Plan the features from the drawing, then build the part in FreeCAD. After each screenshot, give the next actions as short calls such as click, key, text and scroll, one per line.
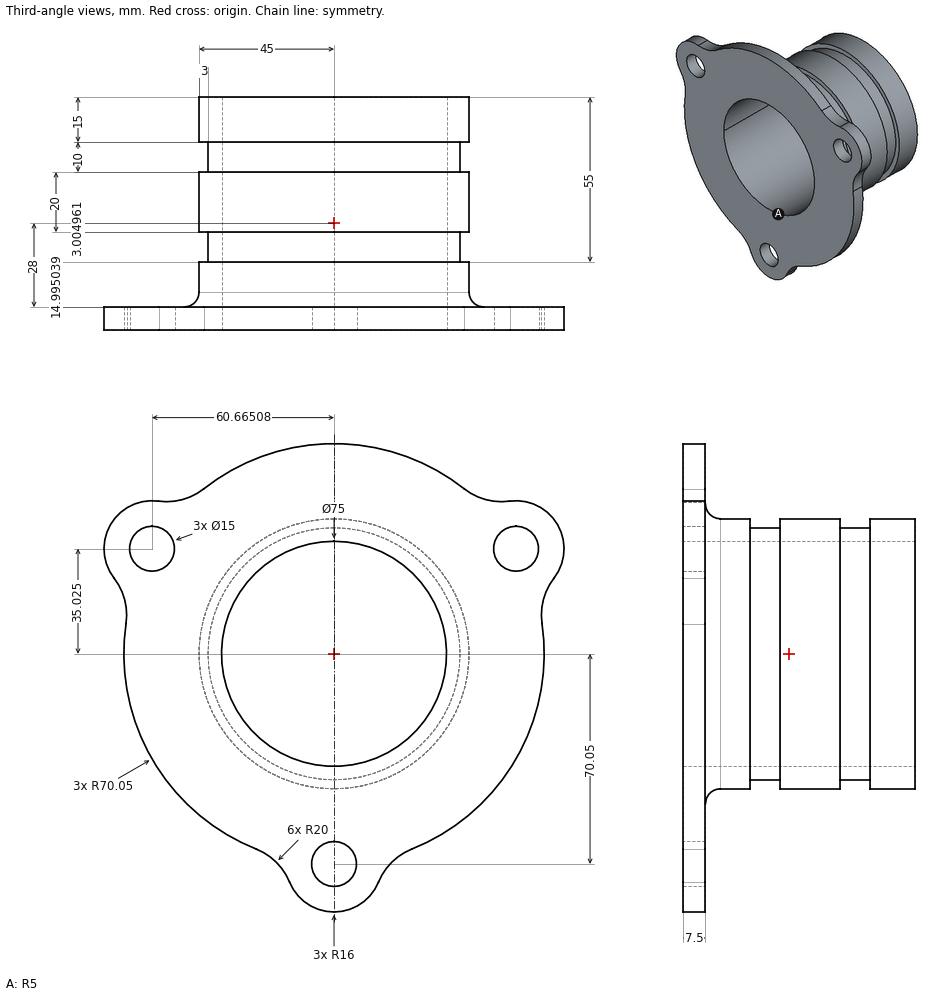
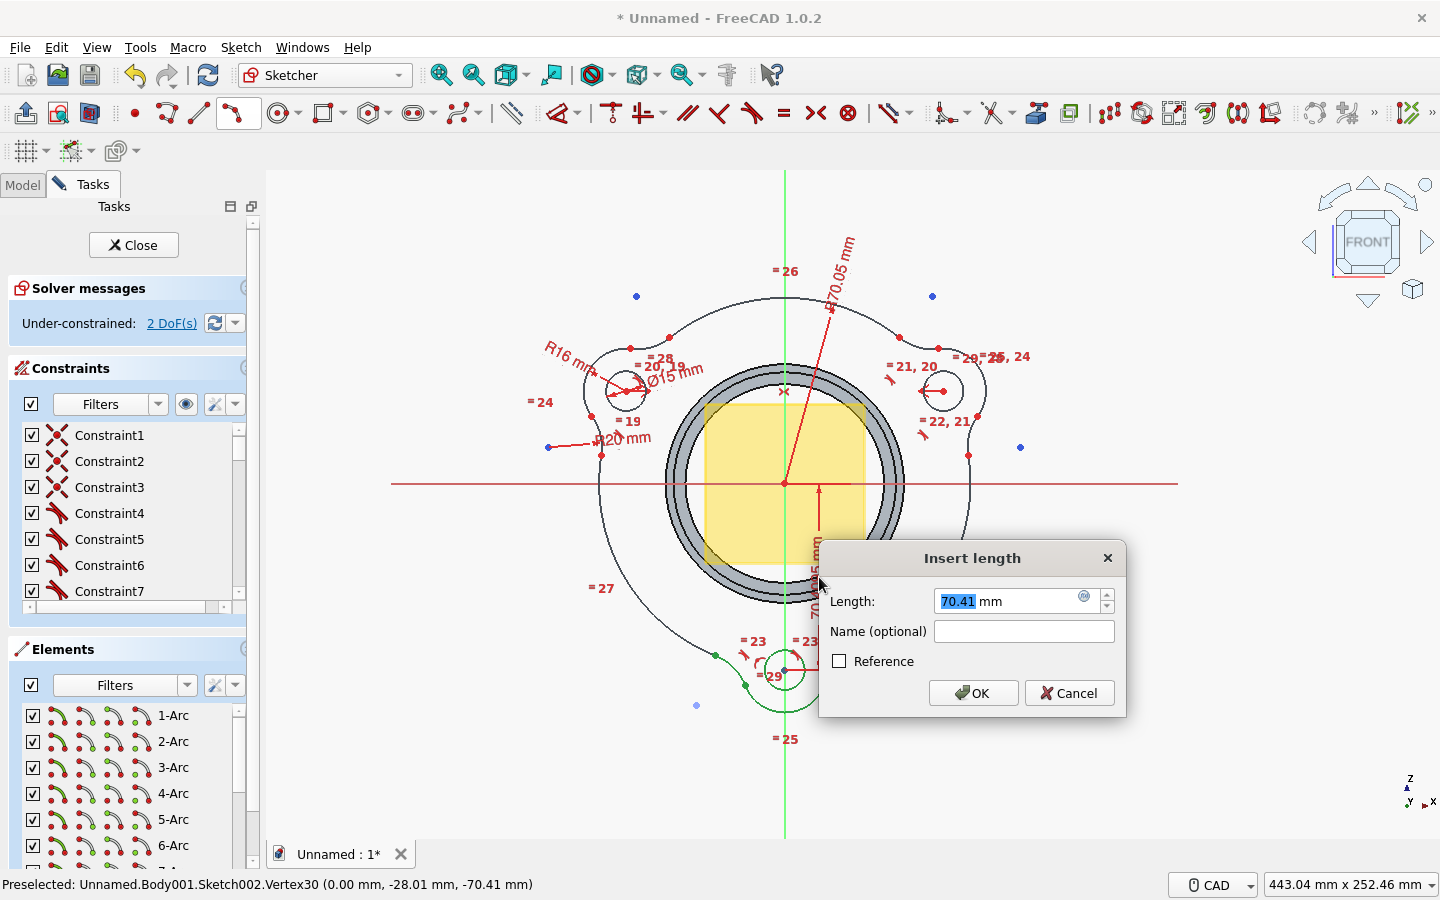
text(70.05)
key(Return)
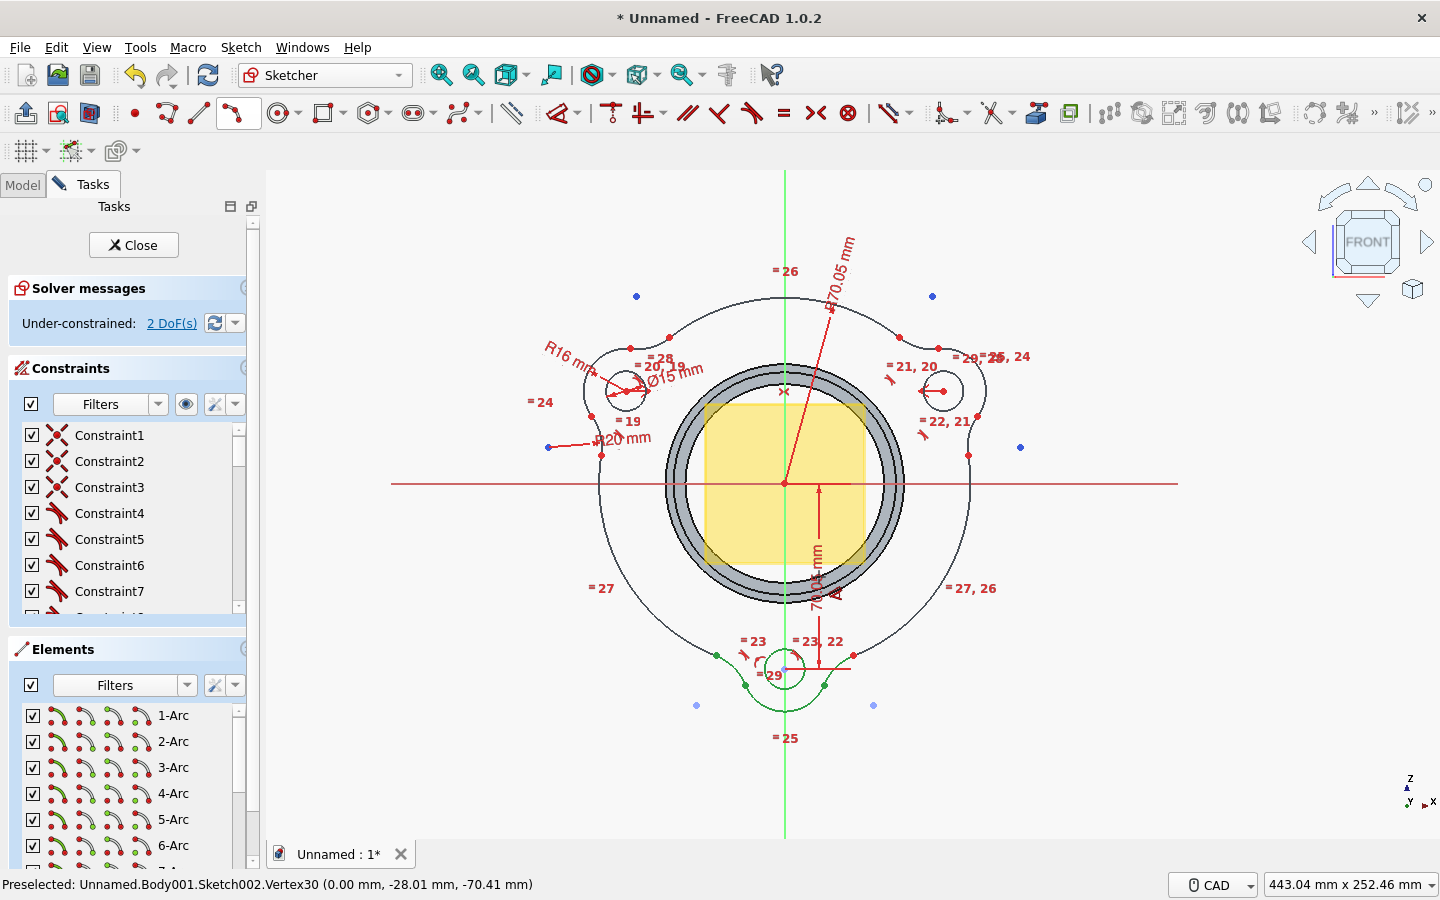
click(626, 391)
click(819, 437)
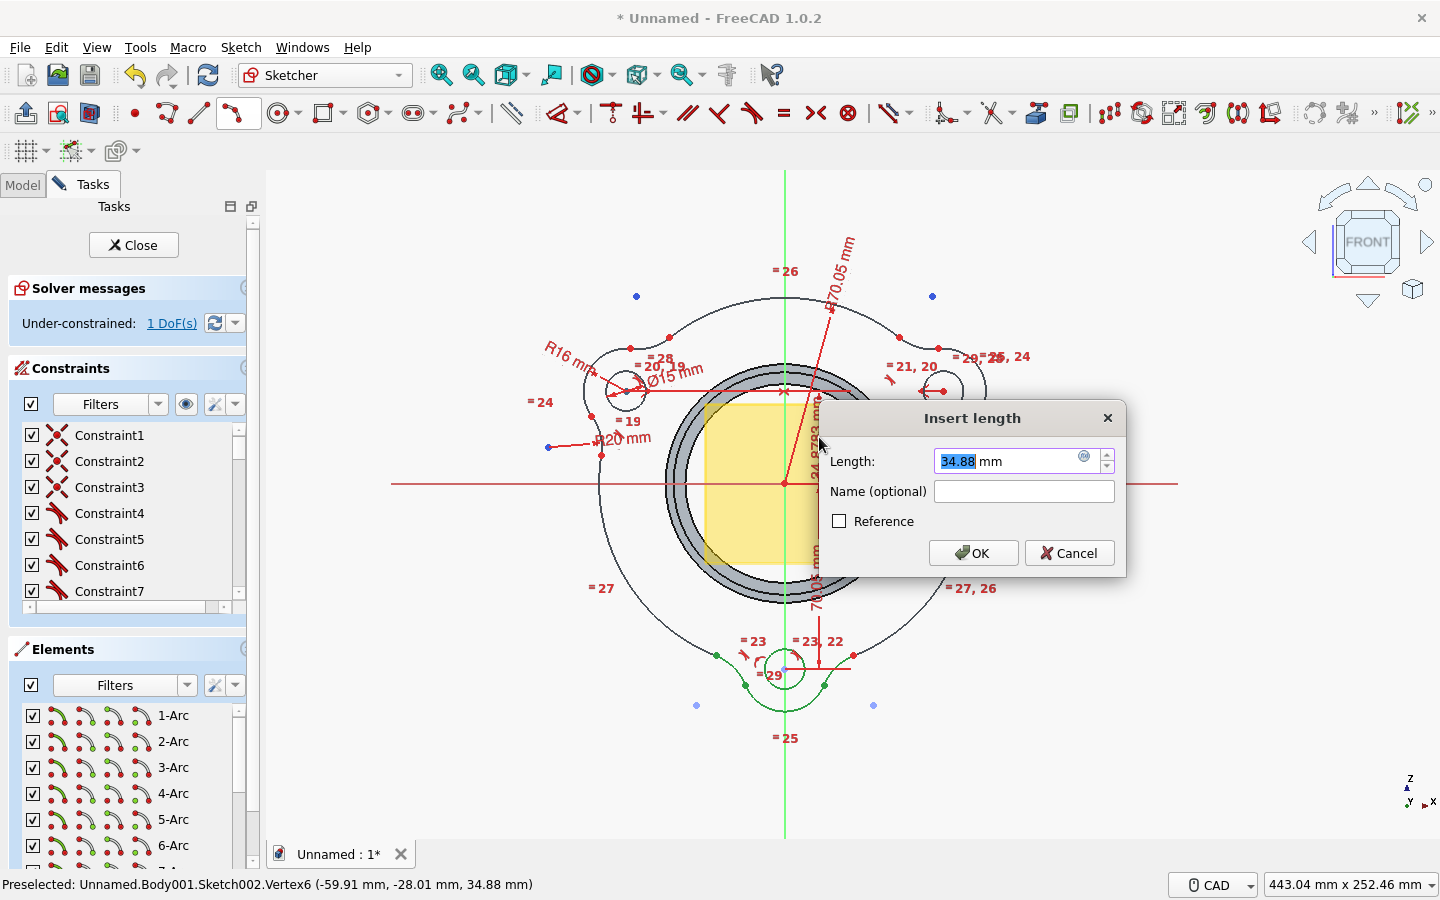
text(35.025)
key(Return)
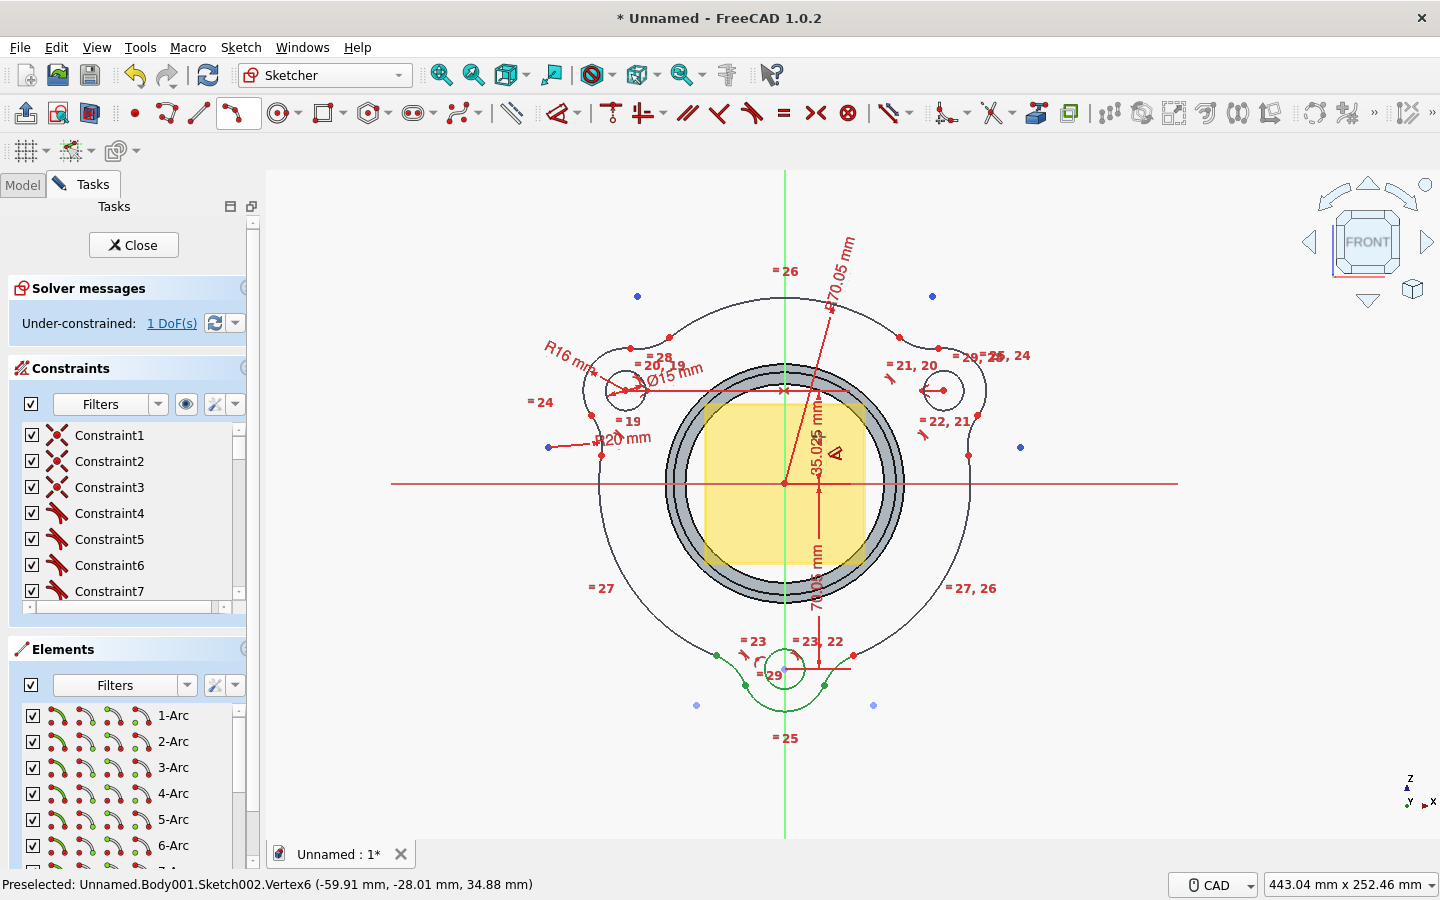
click(626, 391)
click(761, 357)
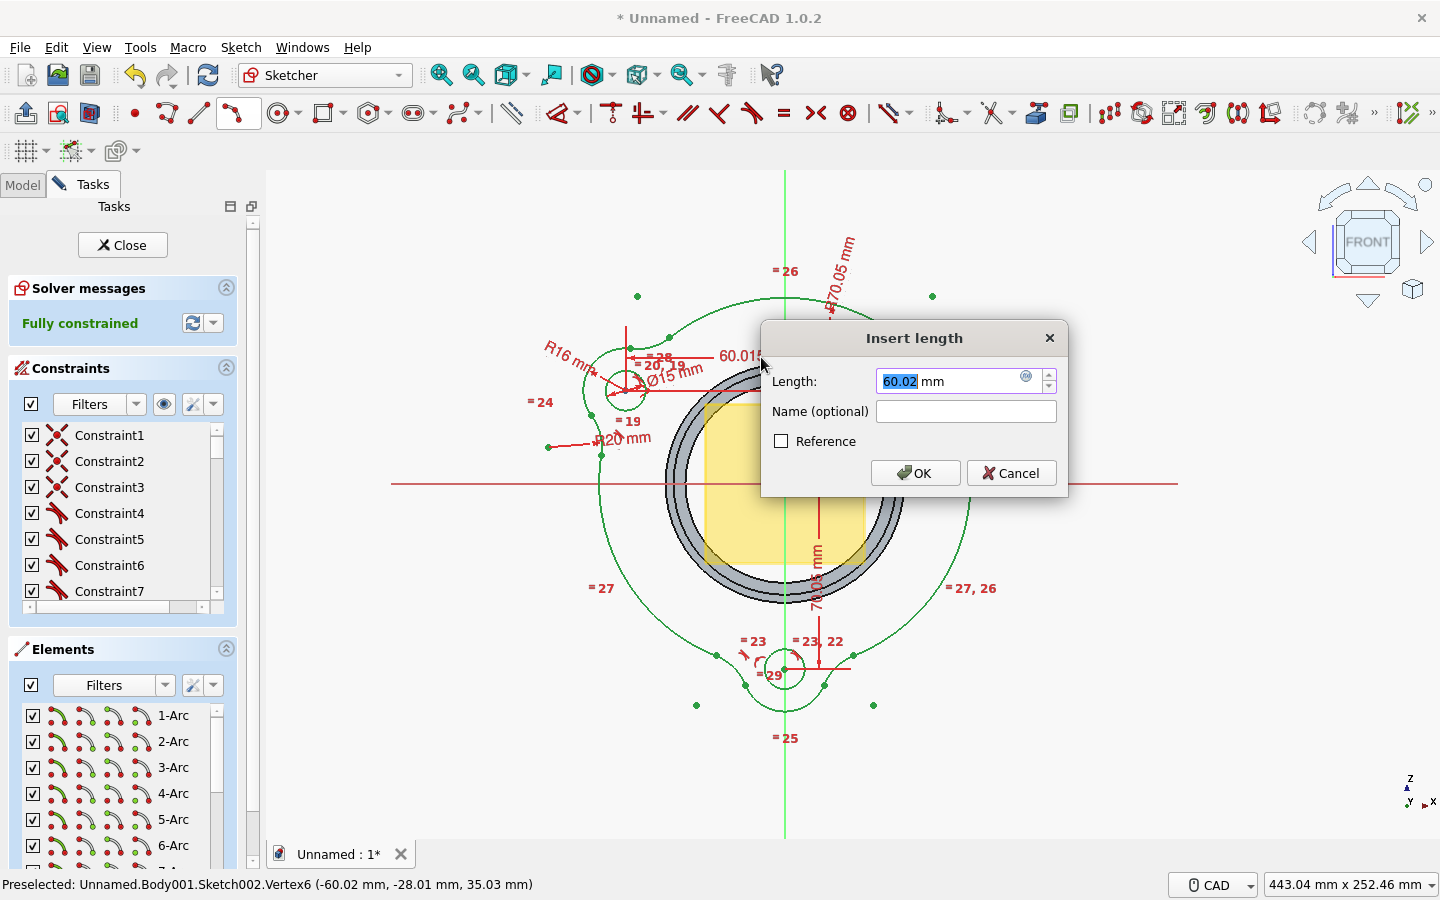
text(60.66508)
key(Return)
key(Escape)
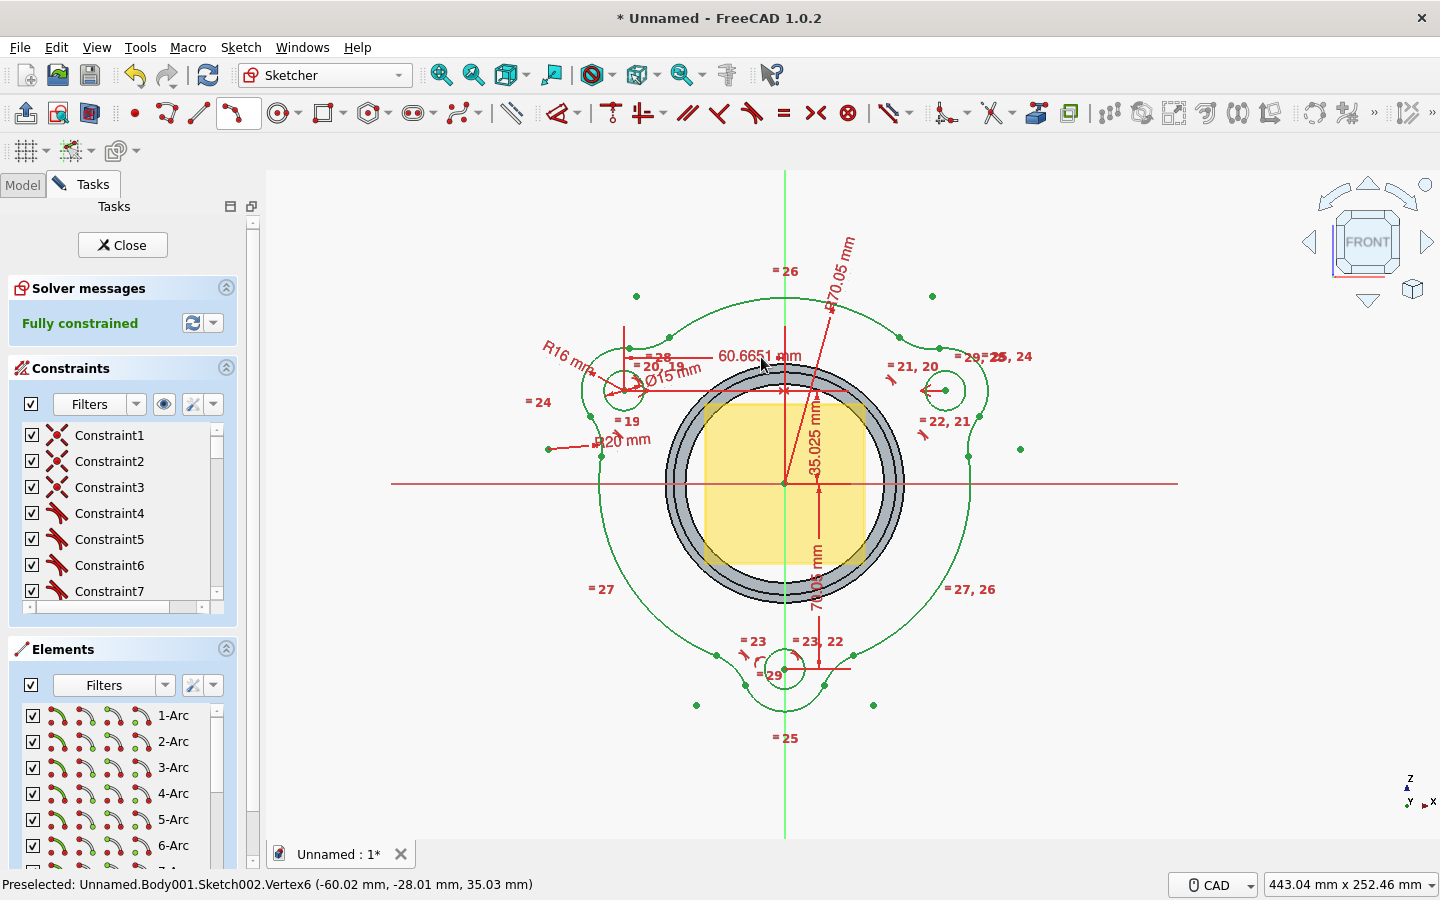
click(123, 245)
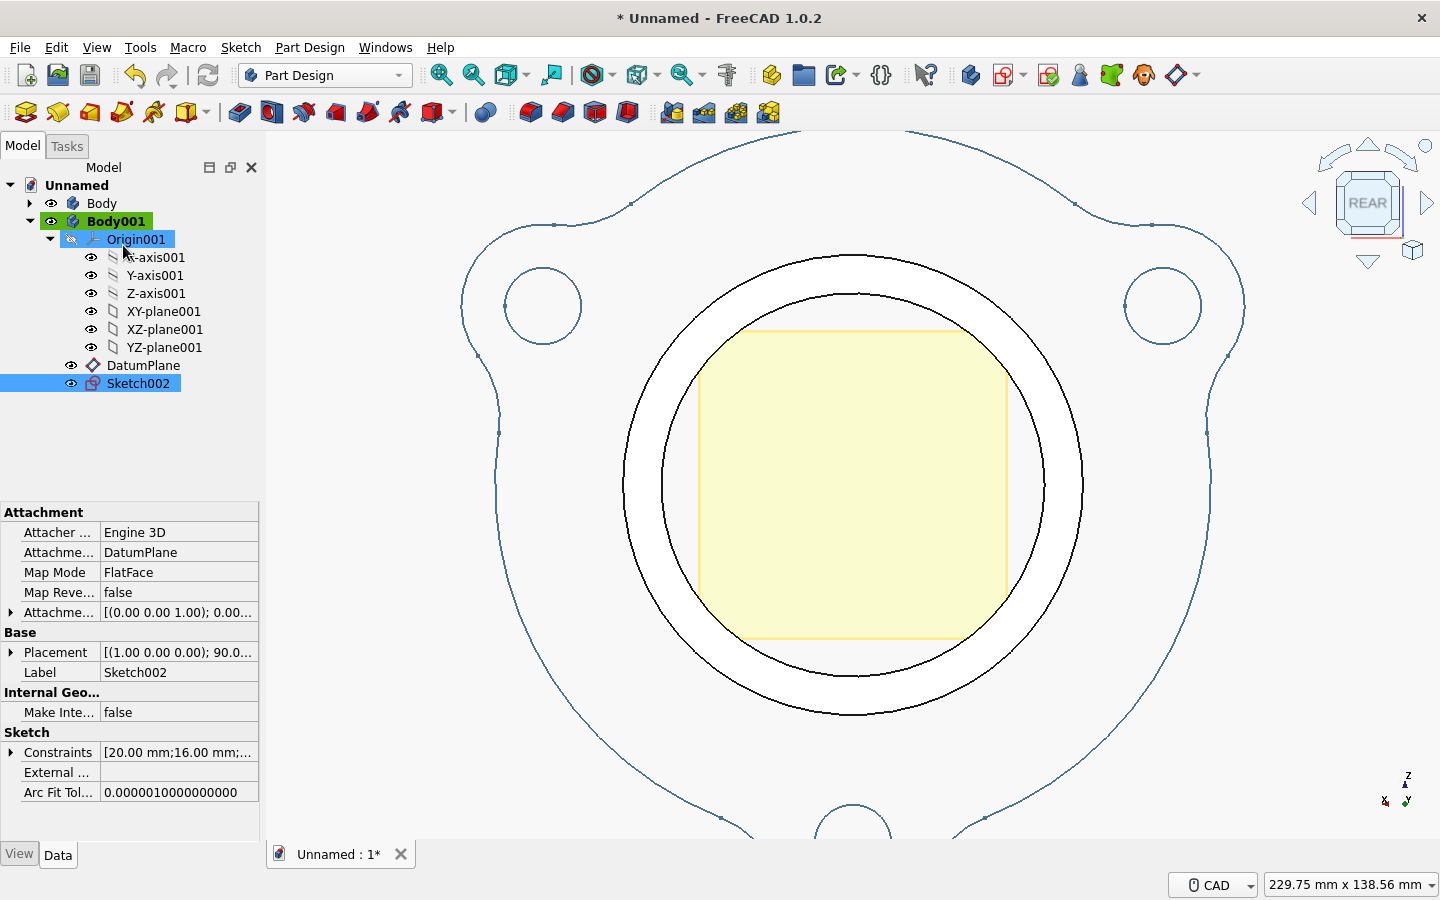
click(26, 112)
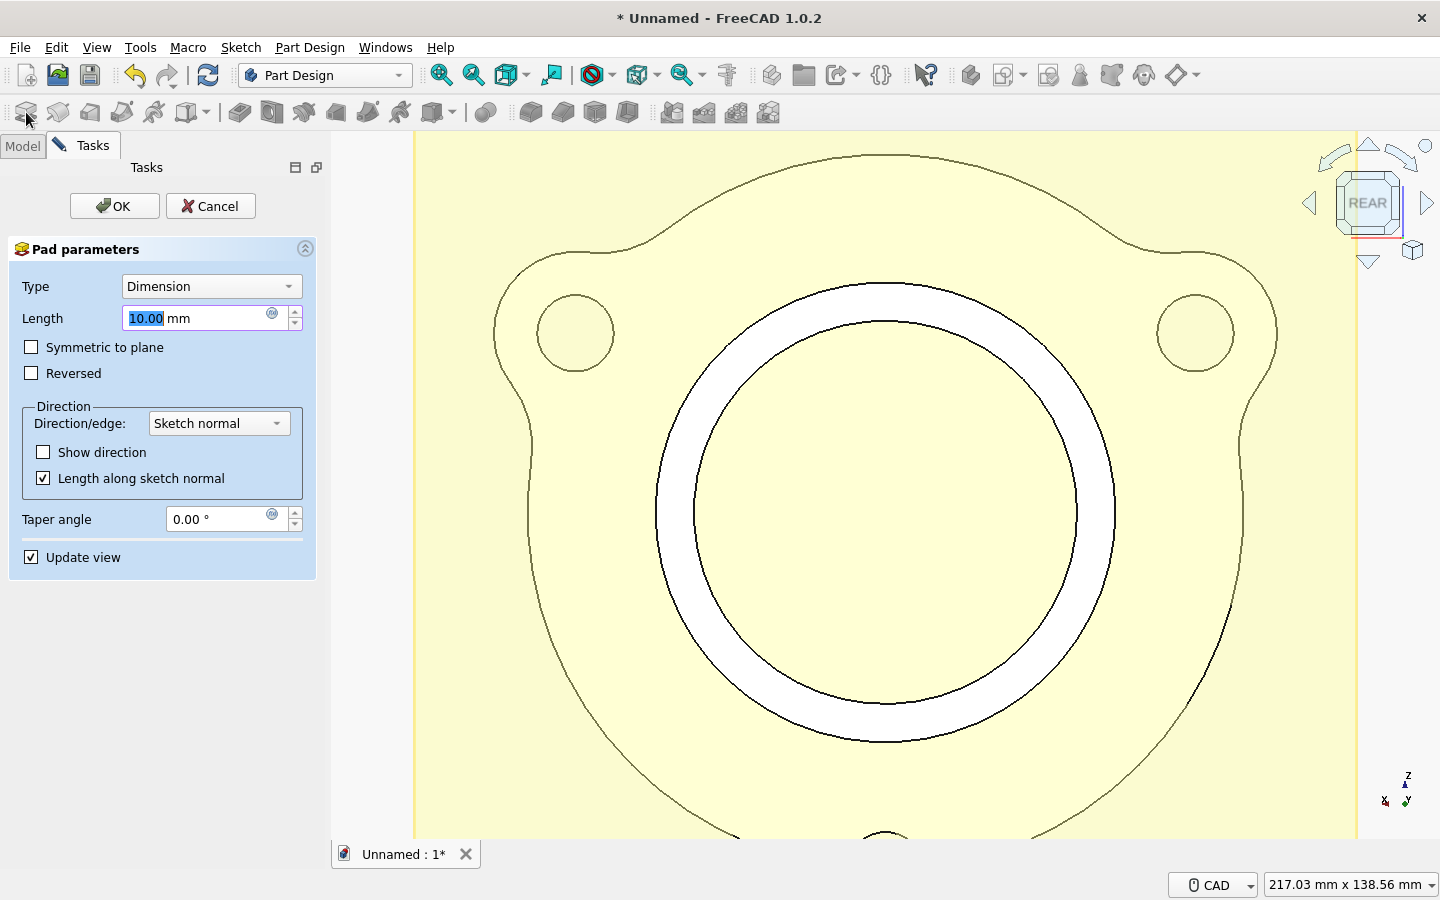
text(7.5)
key(Tab)